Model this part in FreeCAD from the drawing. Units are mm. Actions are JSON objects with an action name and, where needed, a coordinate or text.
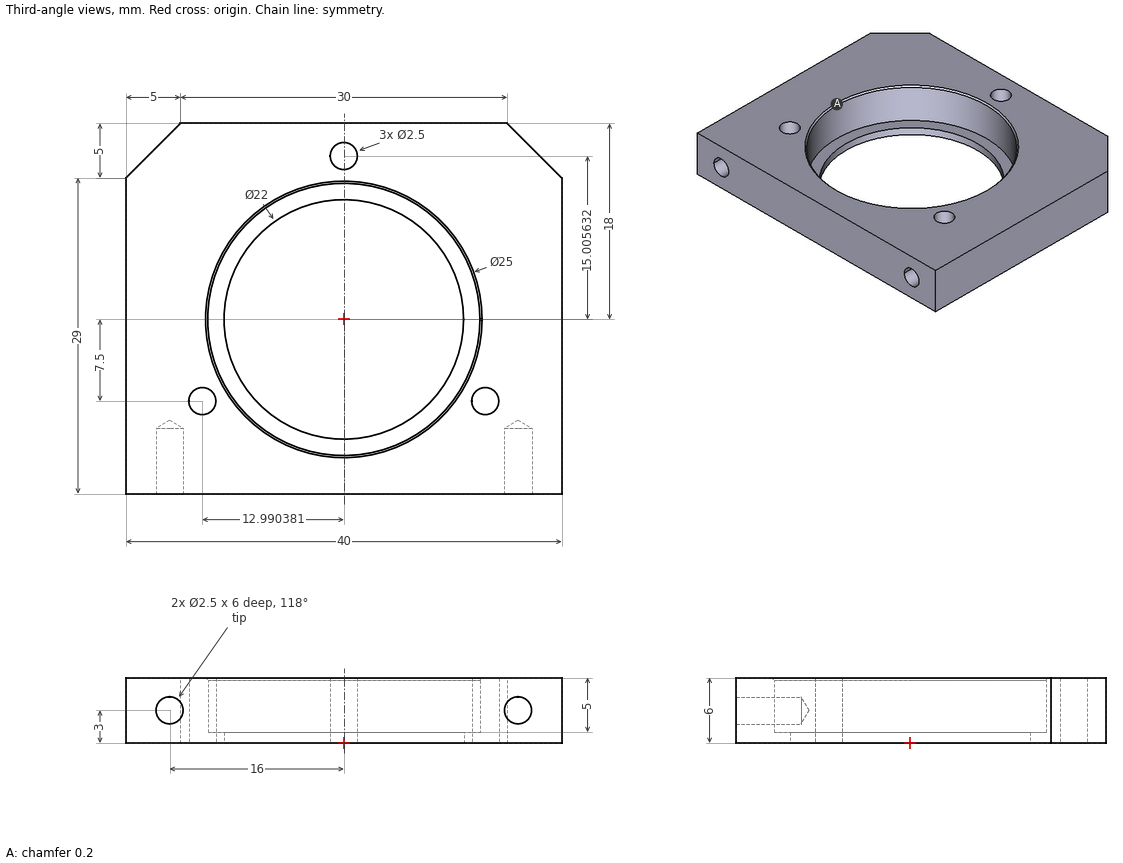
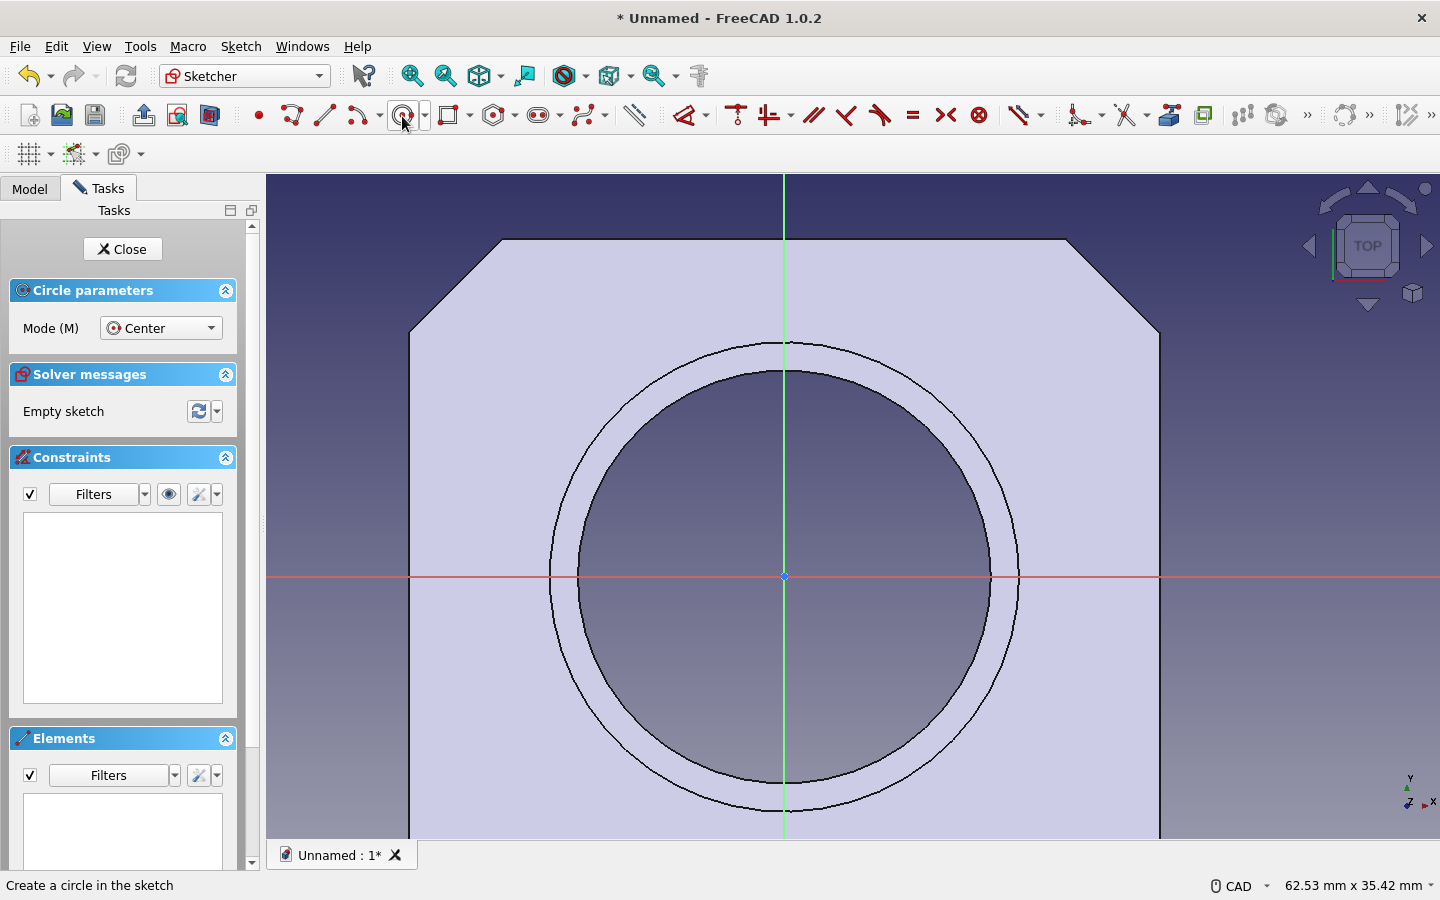
{"action": "left_click", "coordinate": [784, 295]}
{"action": "left_click", "coordinate": [801, 279]}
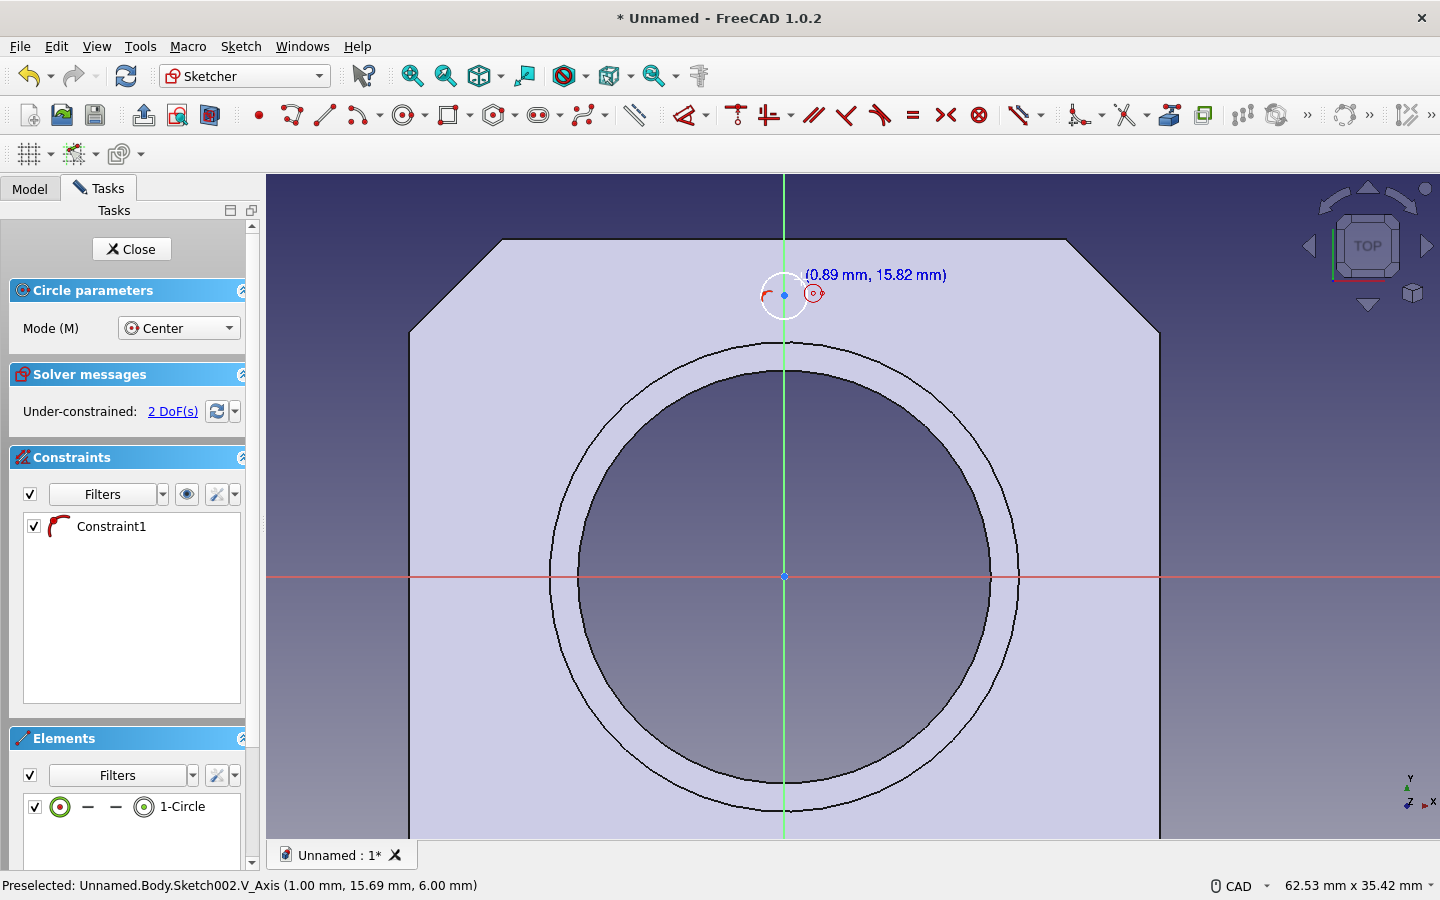
{"action": "left_click", "coordinate": [540, 718]}
{"action": "left_click", "coordinate": [557, 701]}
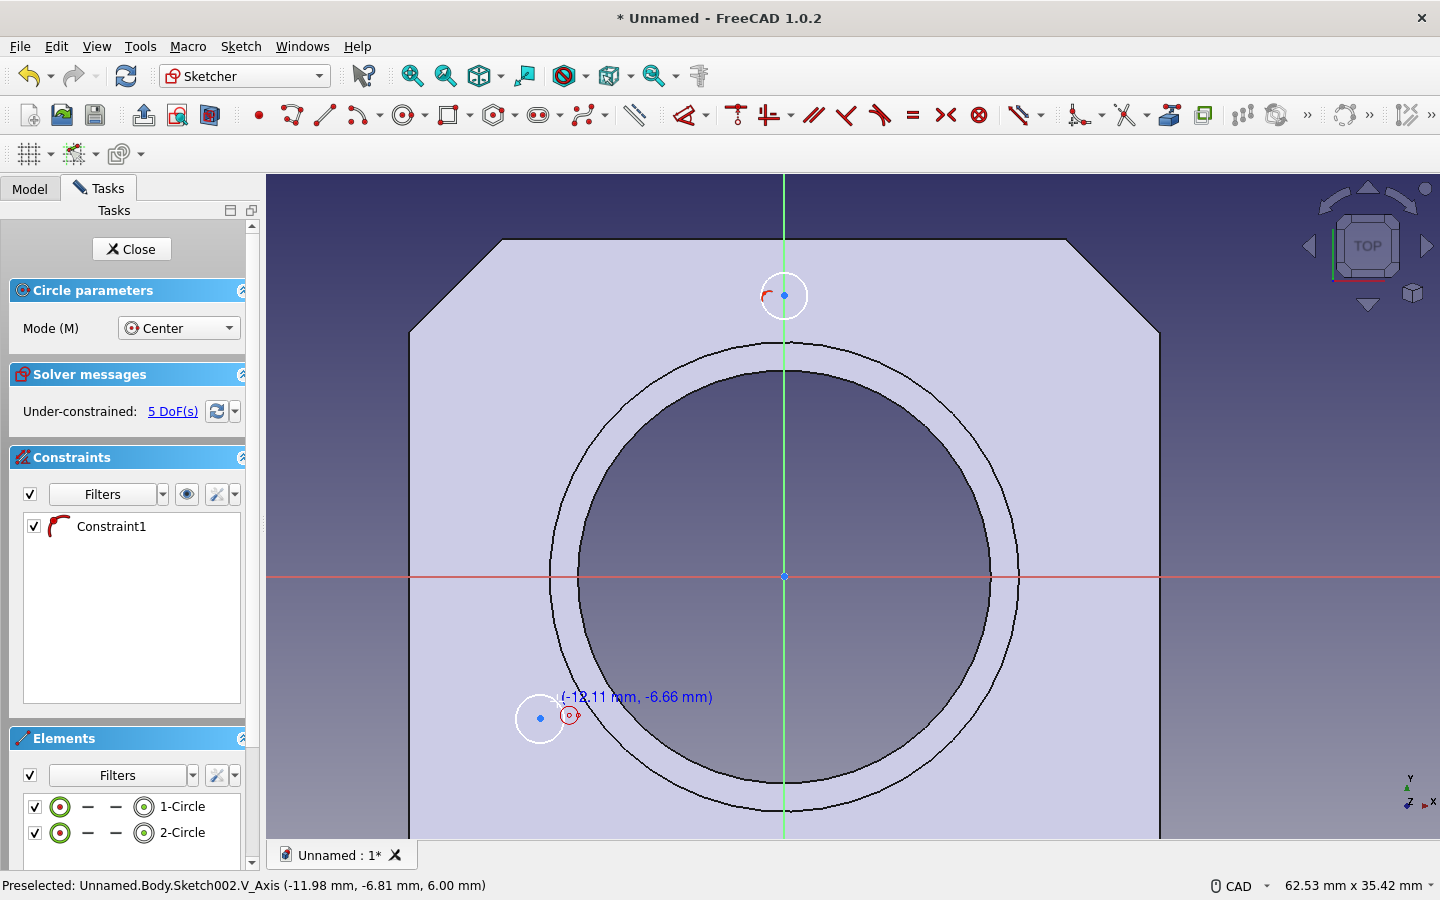
{"action": "left_click", "coordinate": [1028, 718]}
{"action": "left_click", "coordinate": [1045, 701]}
{"action": "key", "text": "Escape"}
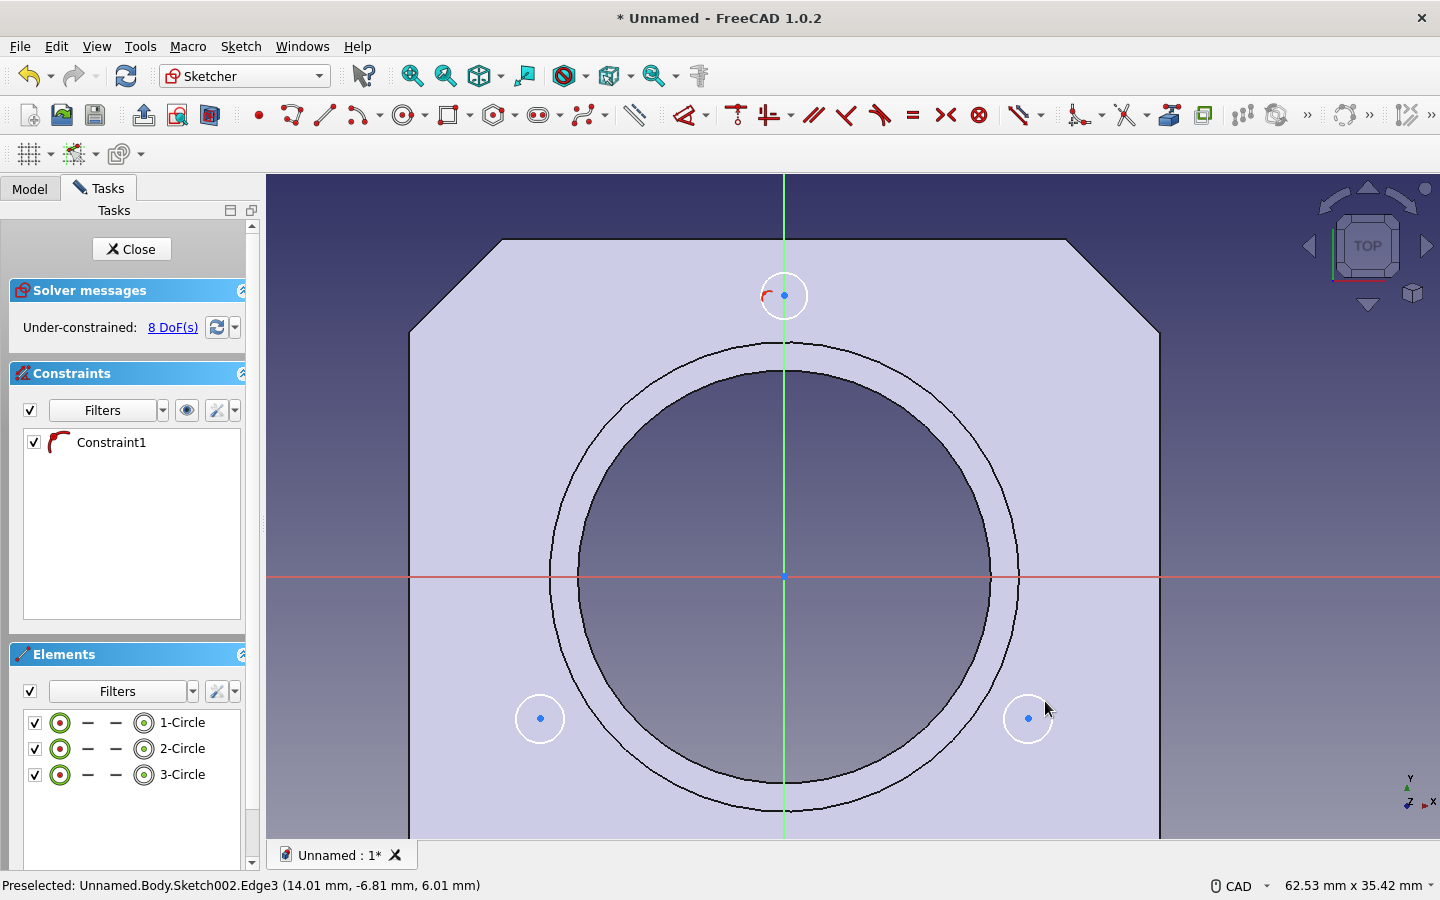
{"action": "left_click", "coordinate": [801, 280]}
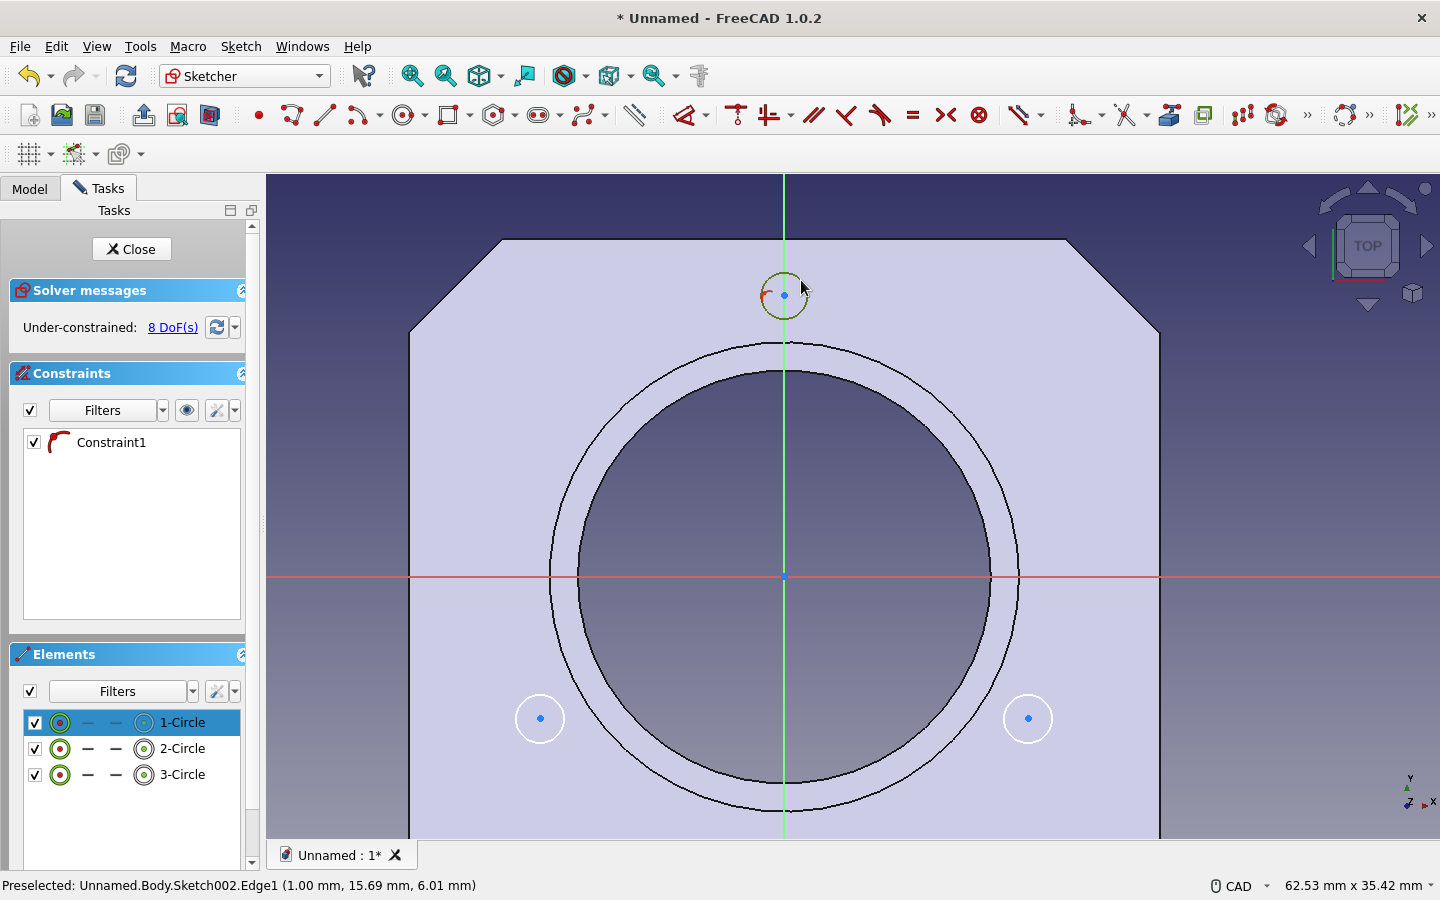
{"action": "left_click", "coordinate": [557, 702]}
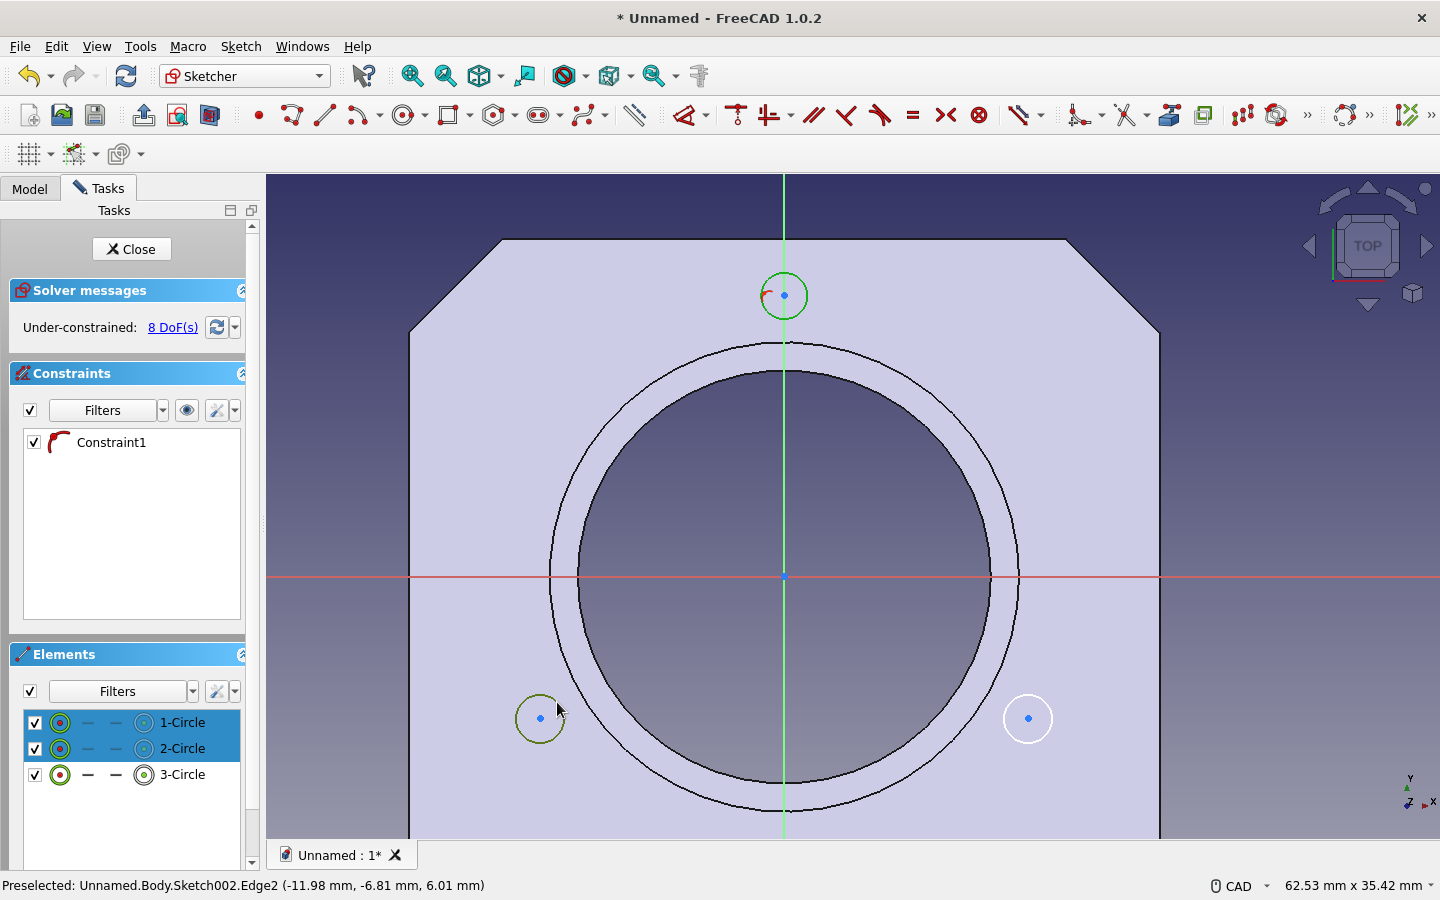
{"action": "left_click", "coordinate": [1045, 702]}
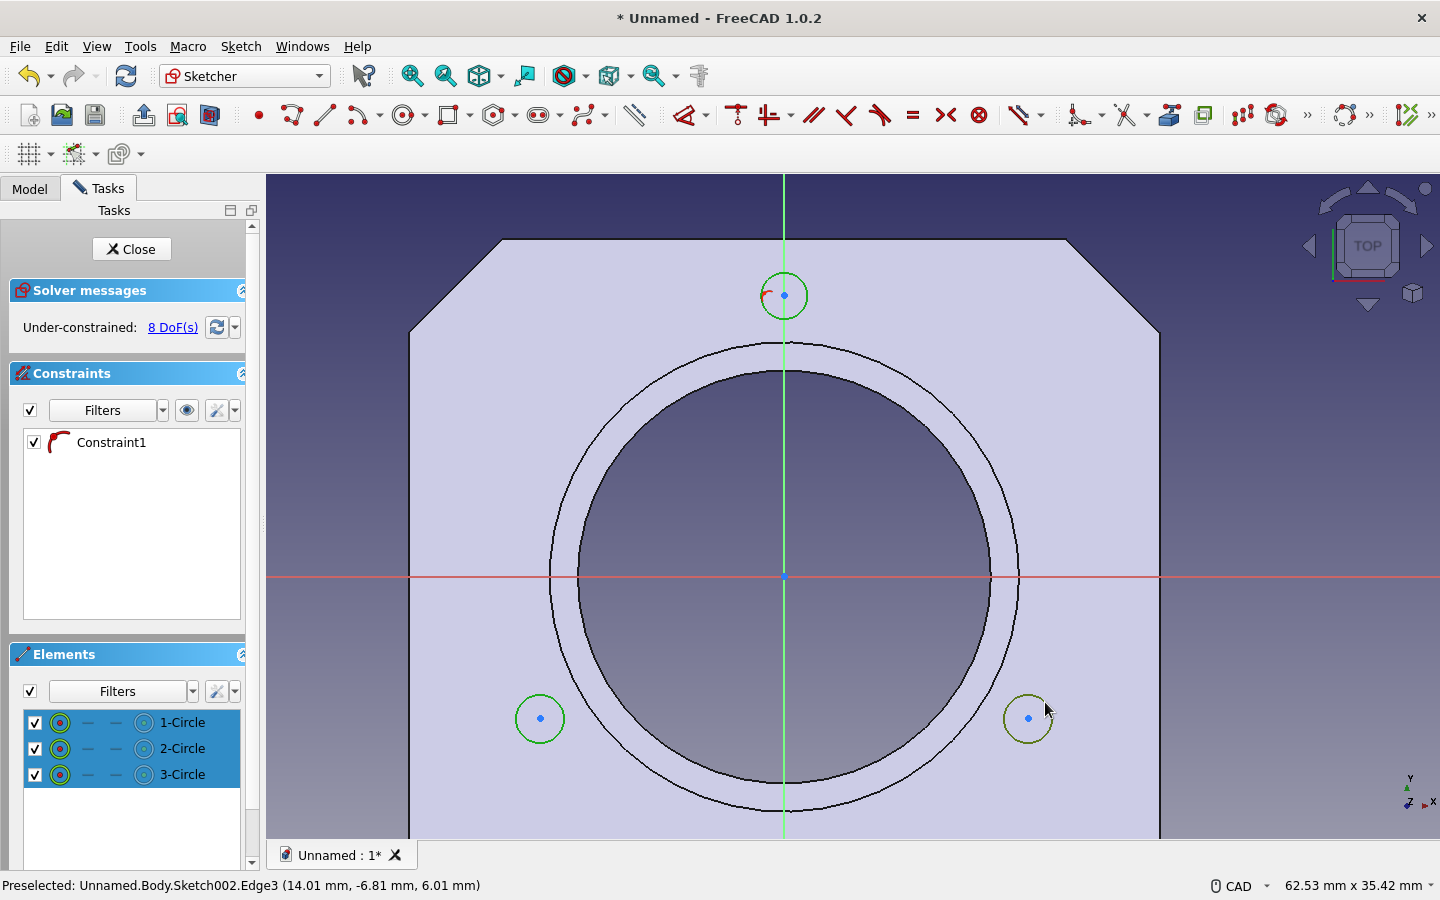
{"action": "left_click", "coordinate": [913, 116]}